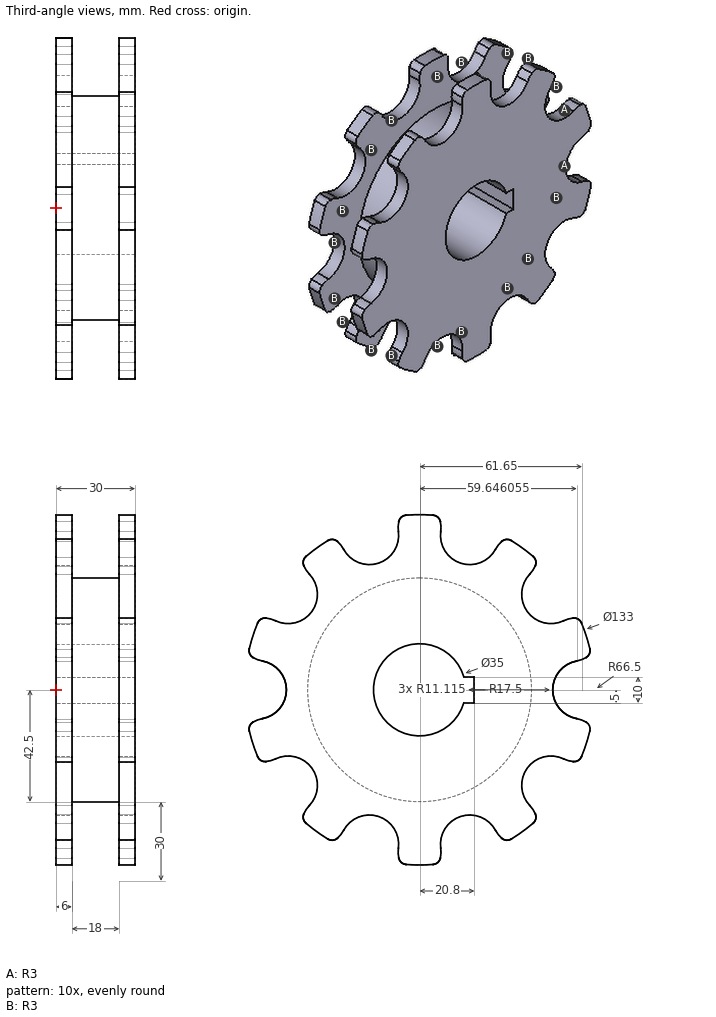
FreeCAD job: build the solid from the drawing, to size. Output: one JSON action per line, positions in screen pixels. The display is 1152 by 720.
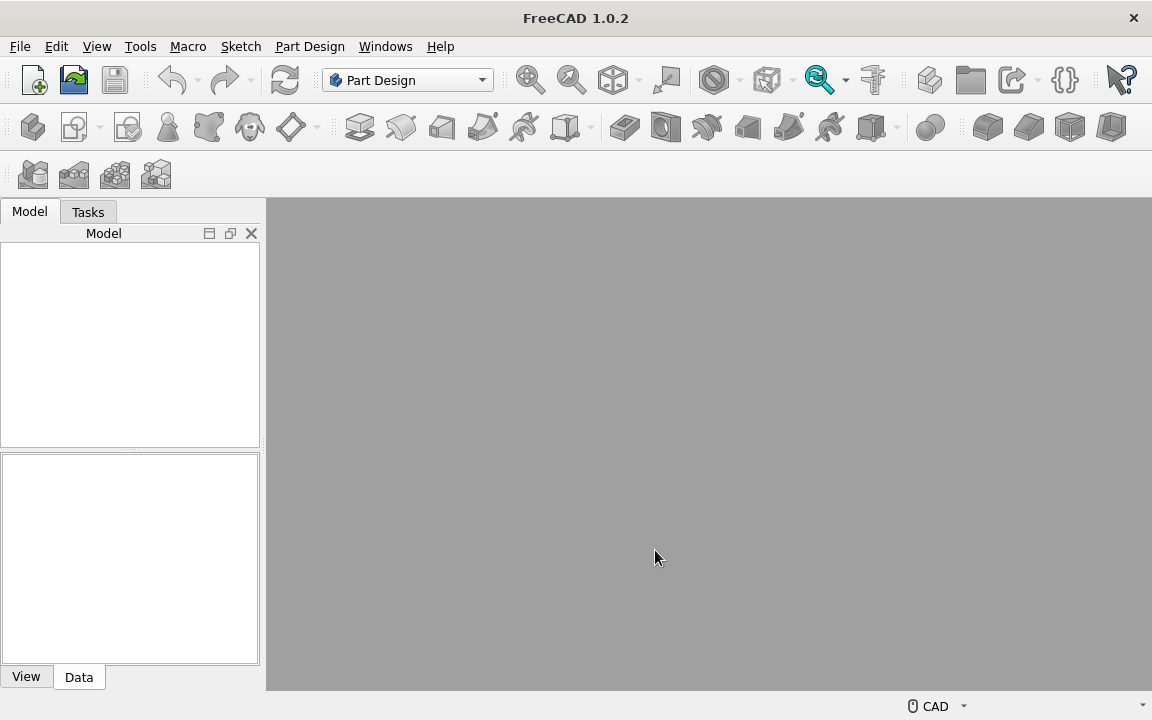
{"action": "left_click", "coordinate": [33, 80]}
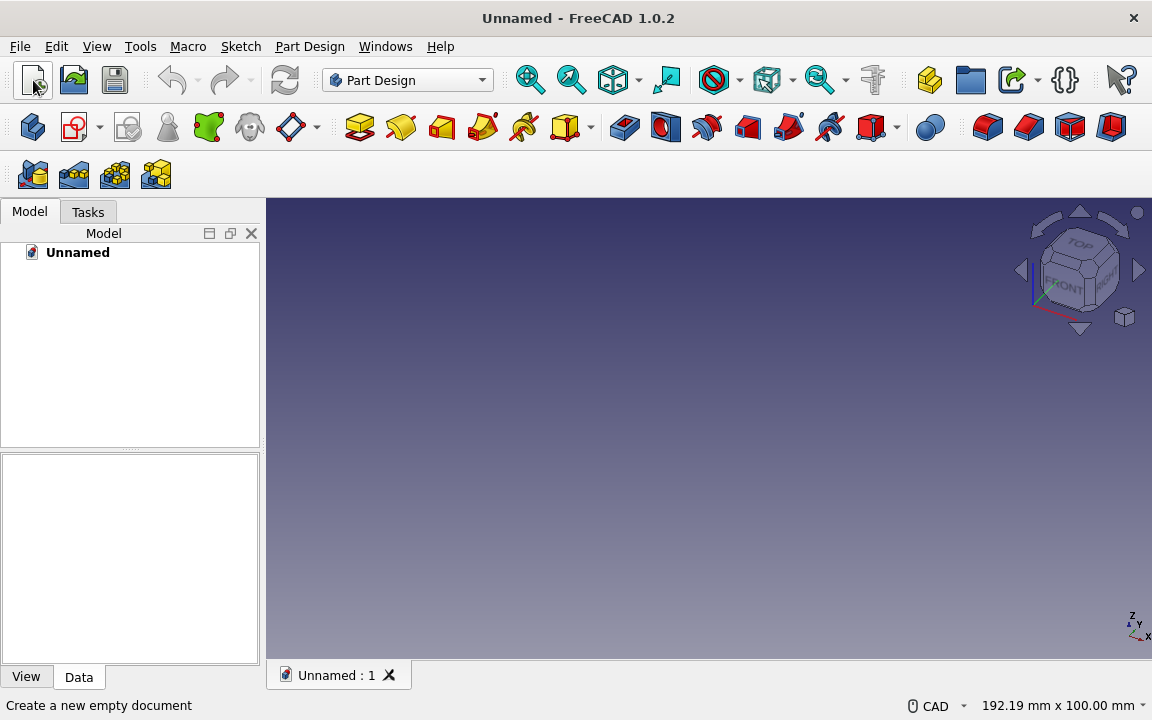
{"action": "left_click", "coordinate": [74, 128]}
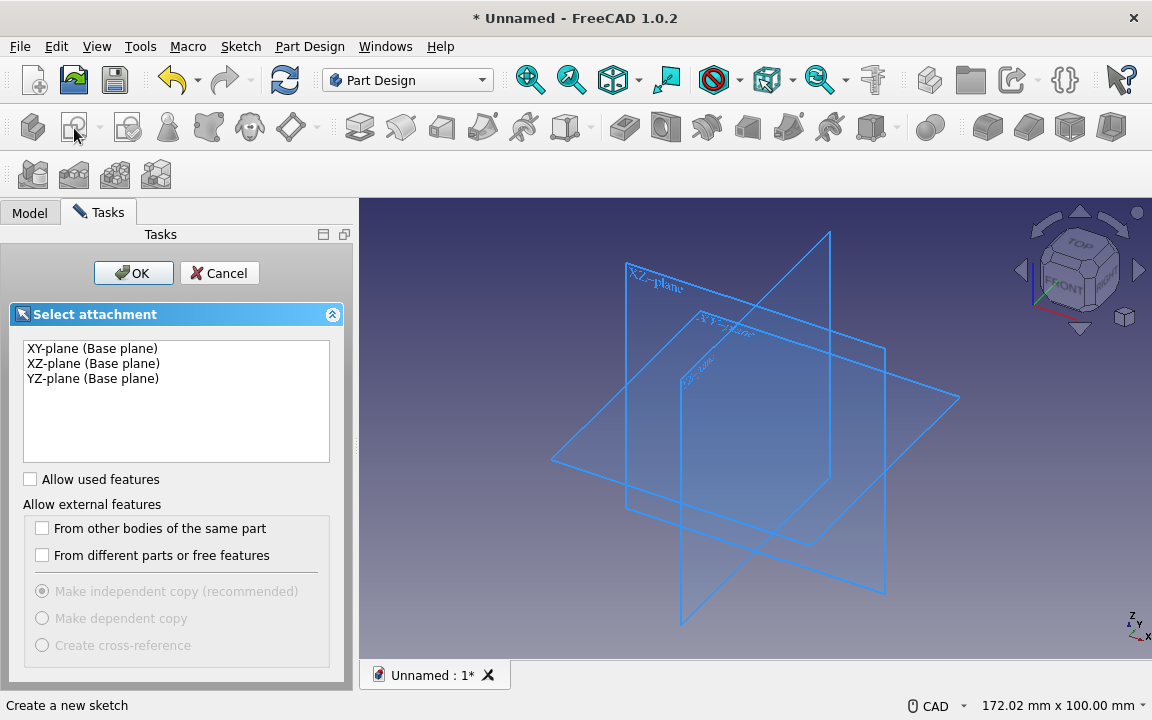
{"action": "left_click", "coordinate": [84, 378]}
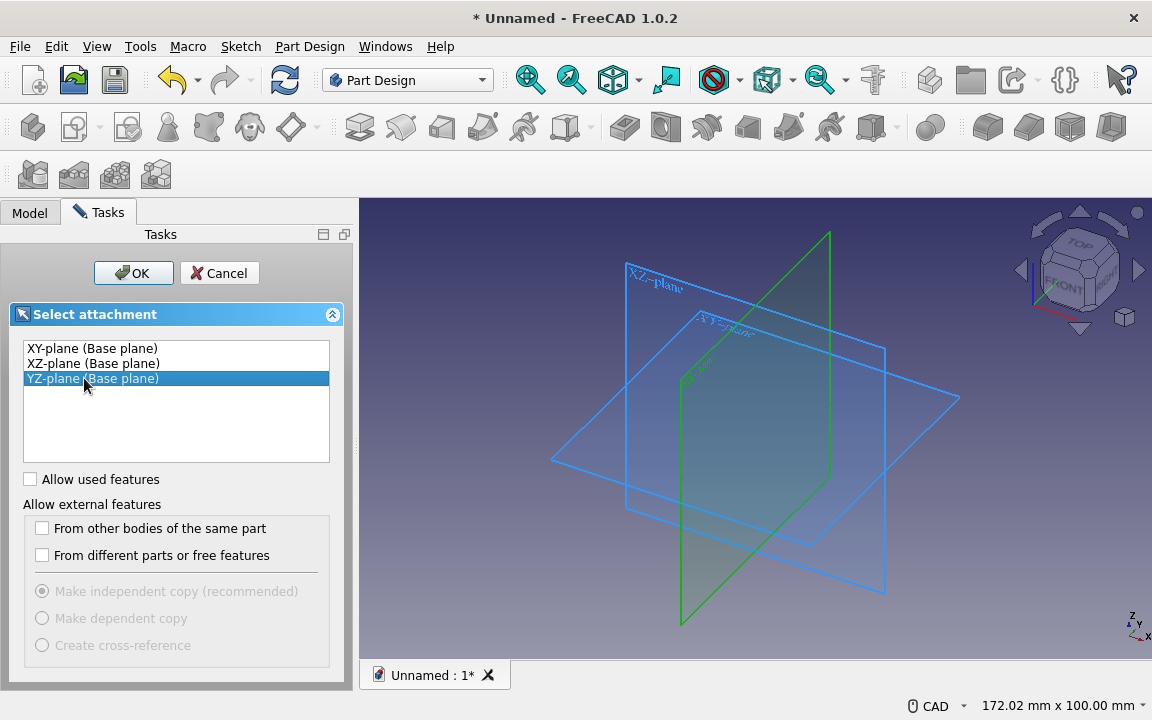
{"action": "left_click", "coordinate": [134, 273]}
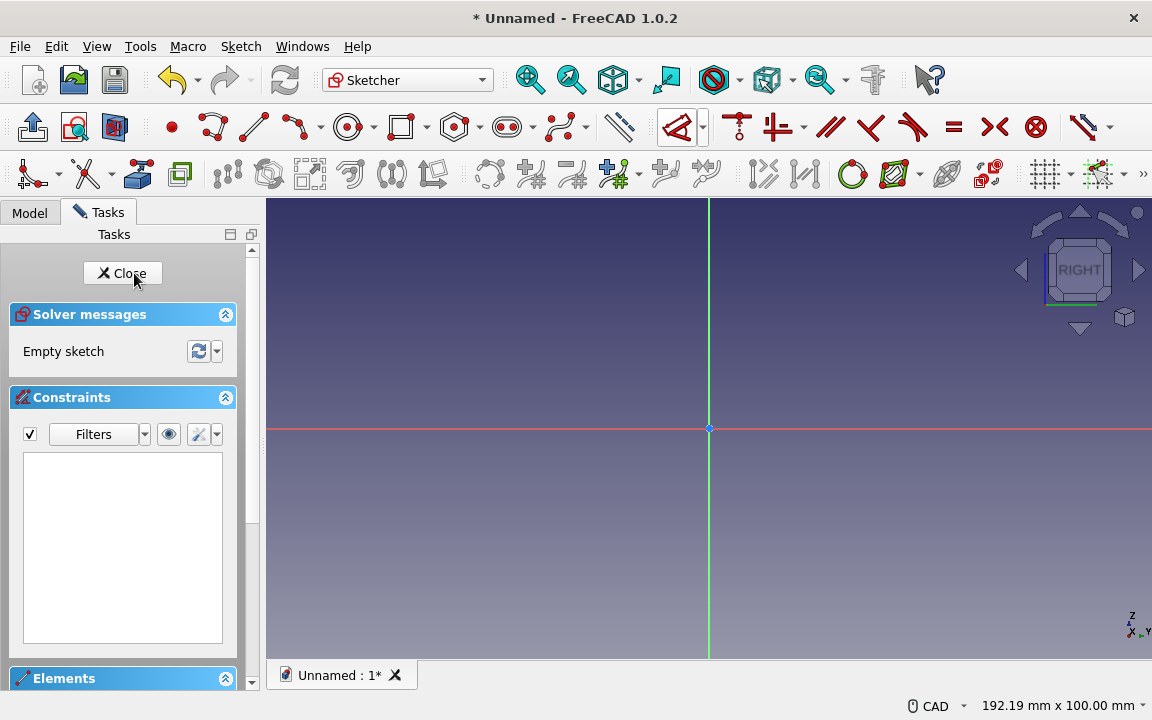
{"action": "scroll", "coordinate": [585, 428], "scroll_direction": "down", "scroll_amount": 4}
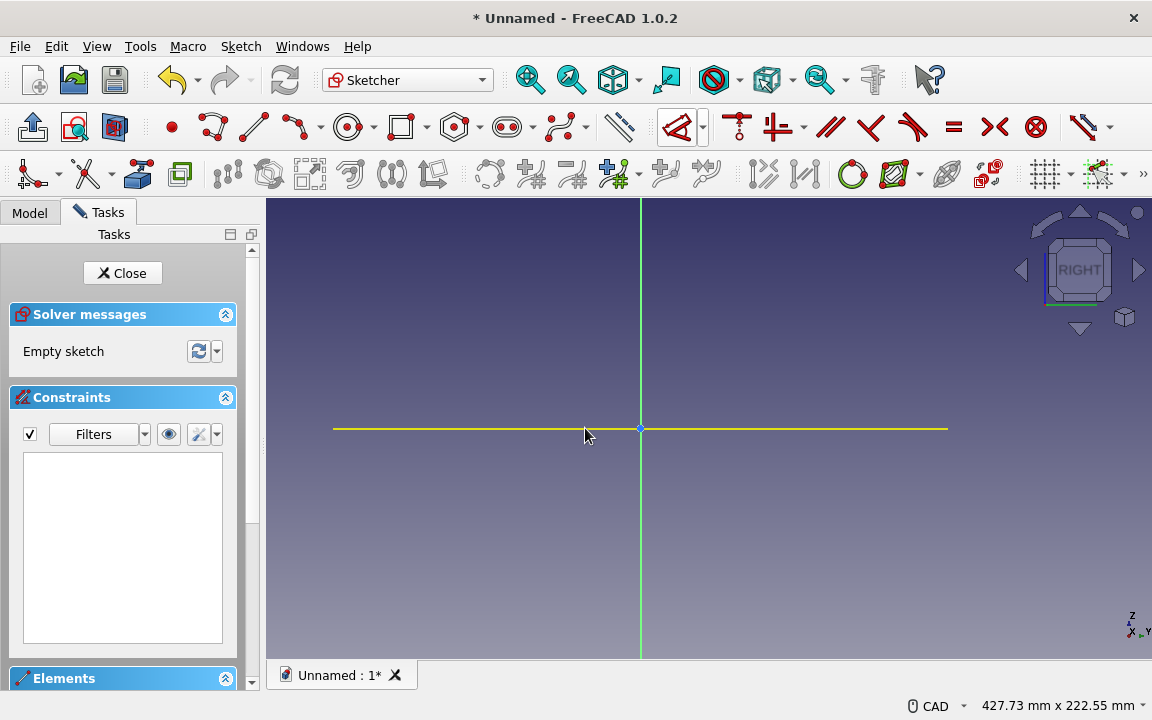
{"action": "left_click", "coordinate": [348, 128]}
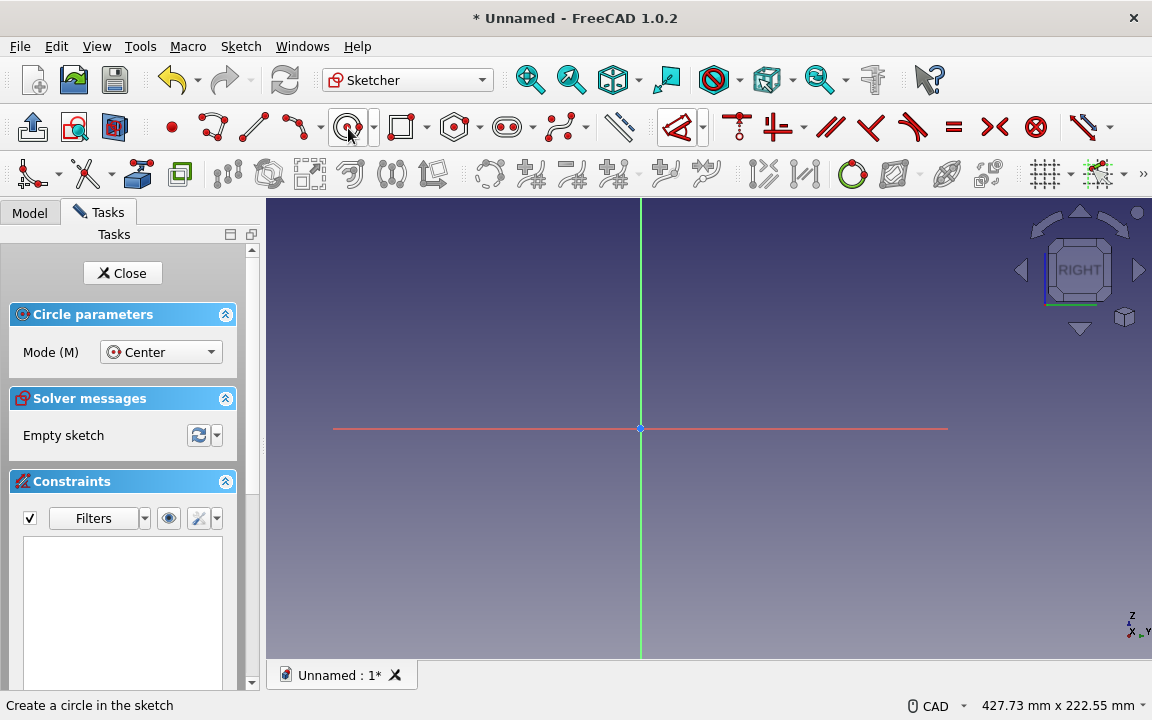
{"action": "left_click", "coordinate": [641, 428]}
{"action": "mouse_move", "coordinate": [738, 331]}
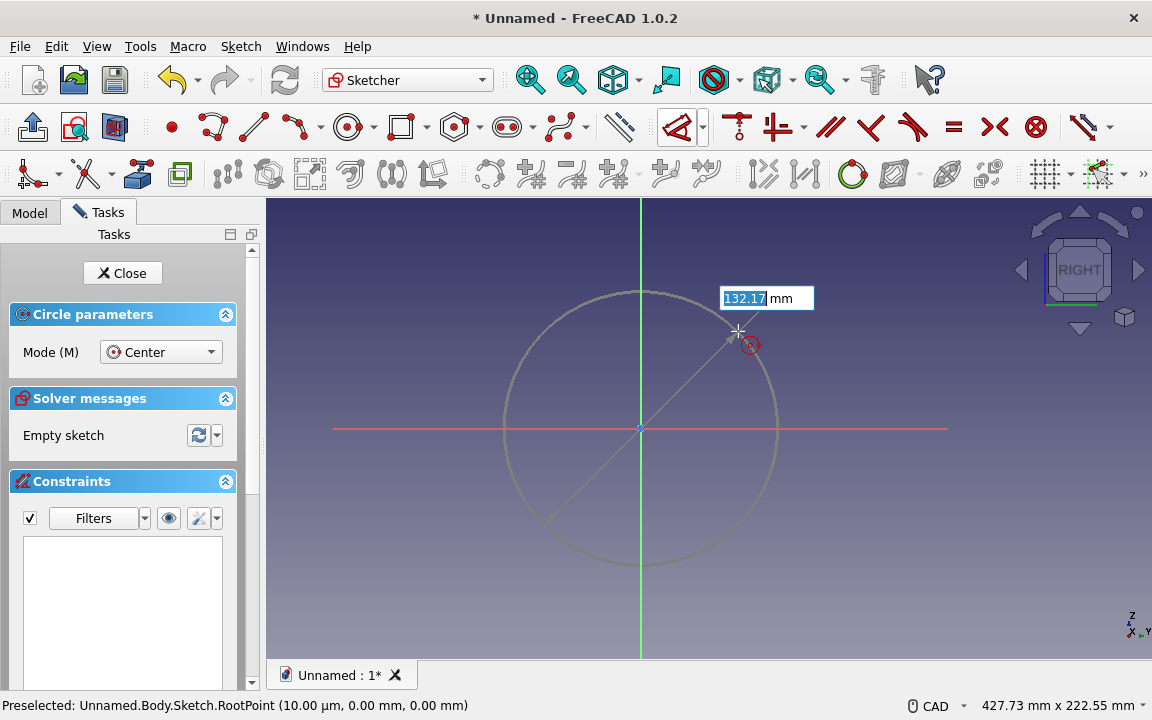
{"action": "type", "text": "133"}
{"action": "key", "text": "Return"}
{"action": "key", "text": "Escape"}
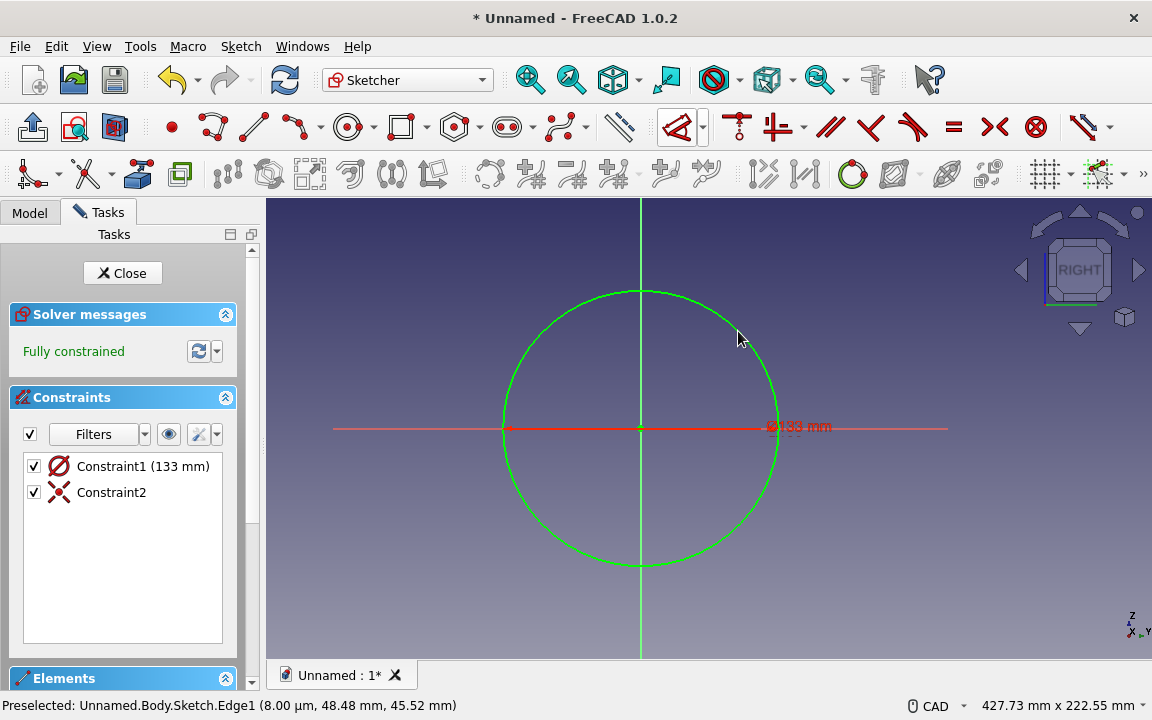
{"action": "left_click", "coordinate": [123, 273]}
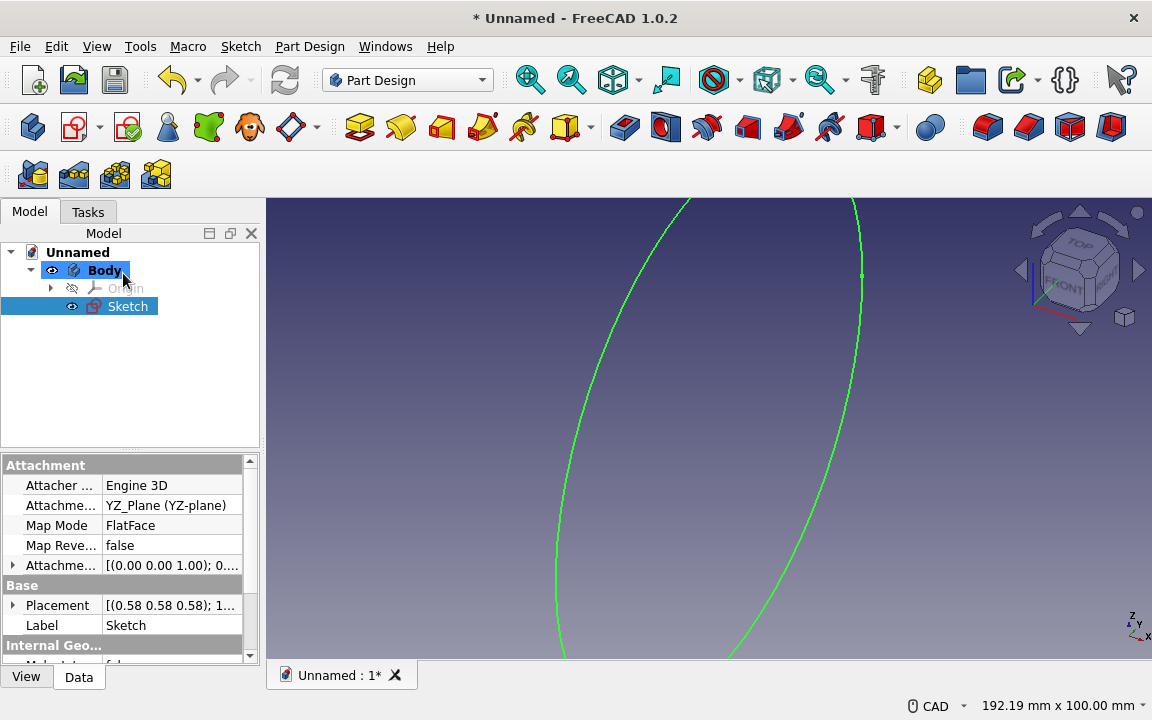
{"action": "left_click", "coordinate": [360, 128]}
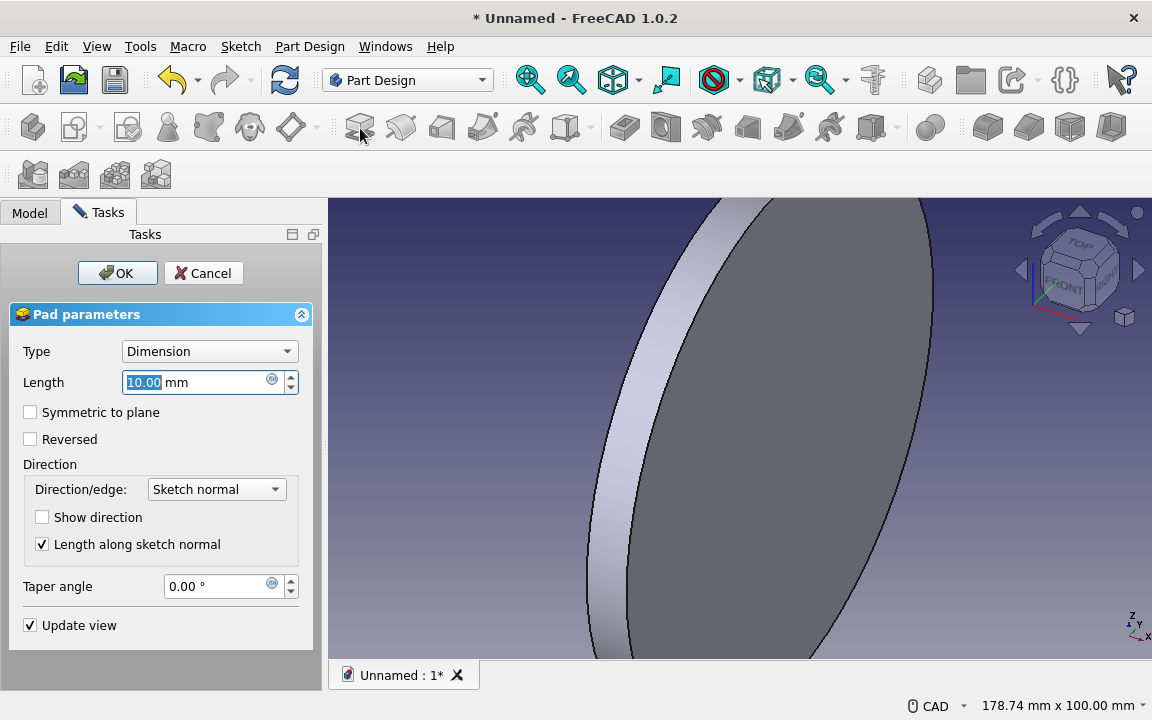
{"action": "type", "text": "30"}
{"action": "key", "text": "Tab"}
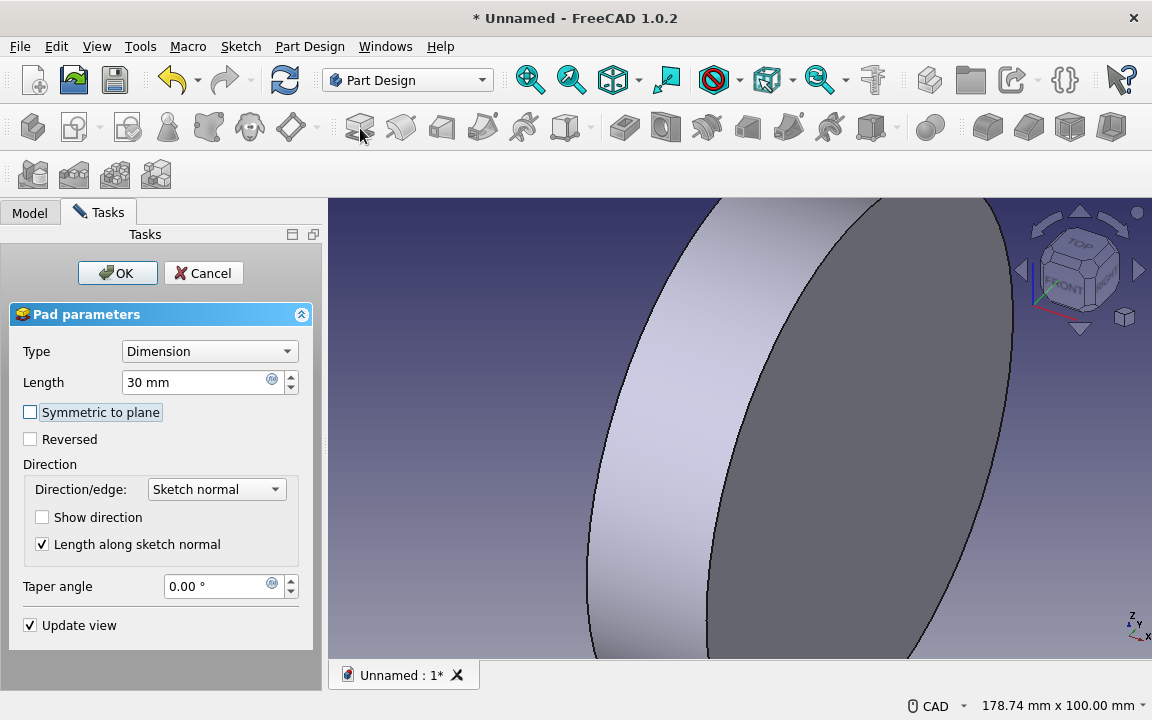
{"action": "left_click", "coordinate": [118, 273]}